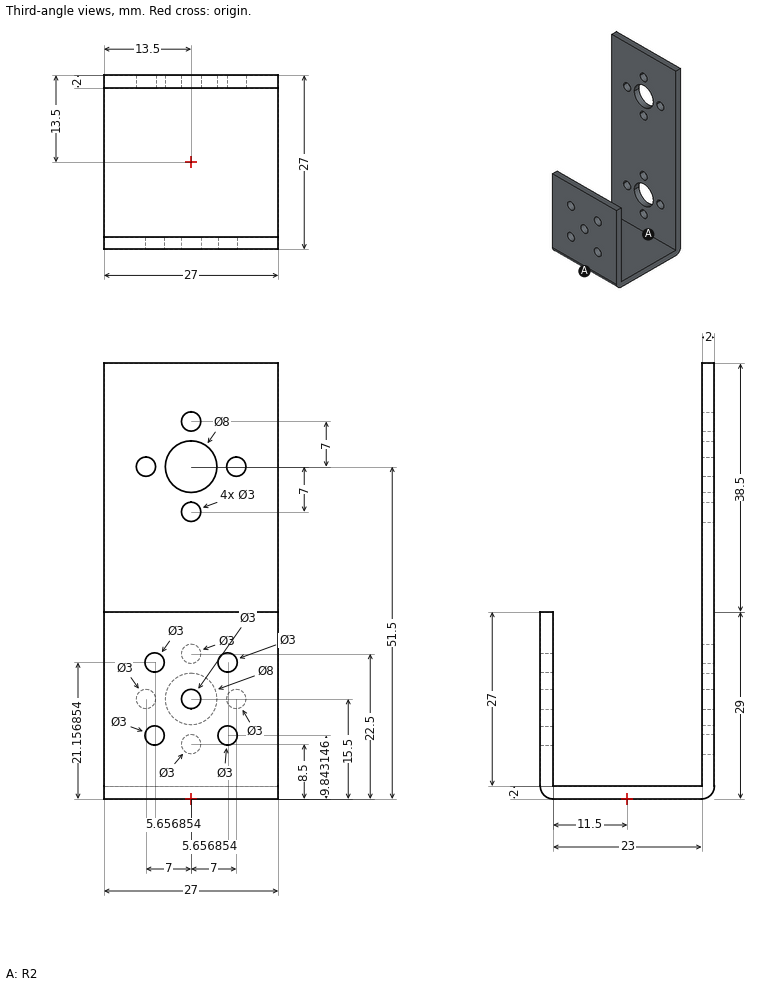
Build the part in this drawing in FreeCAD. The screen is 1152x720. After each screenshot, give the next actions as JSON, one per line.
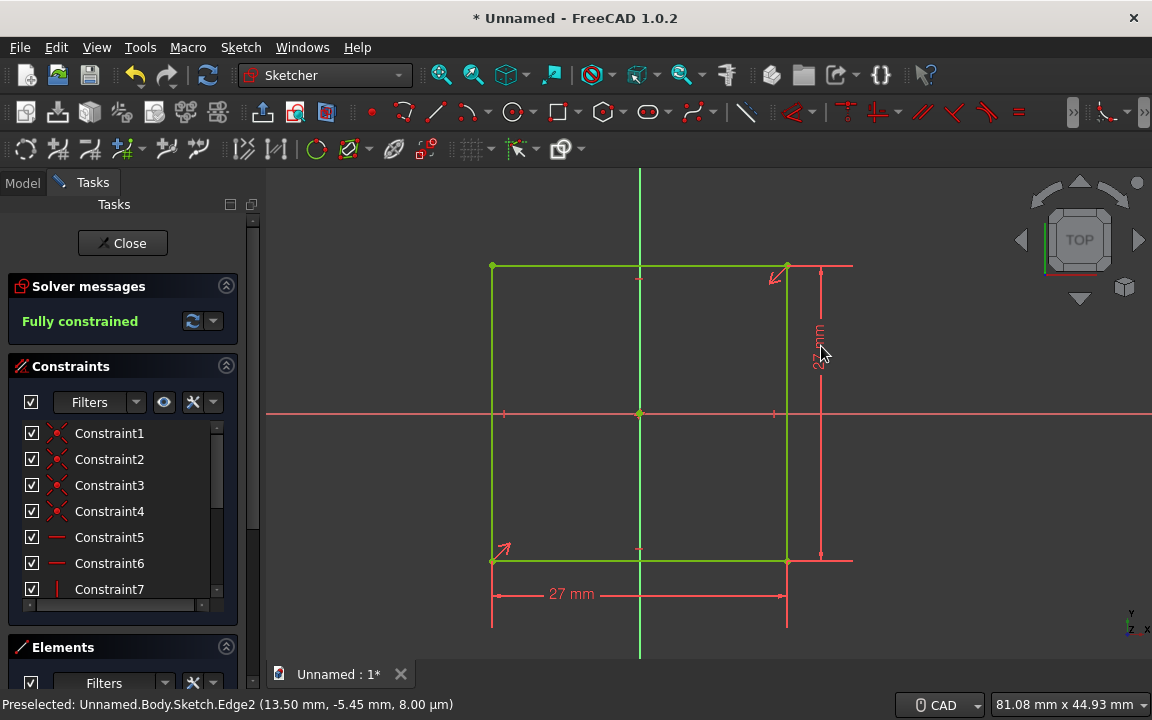
{"action": "left_click", "coordinate": [123, 243]}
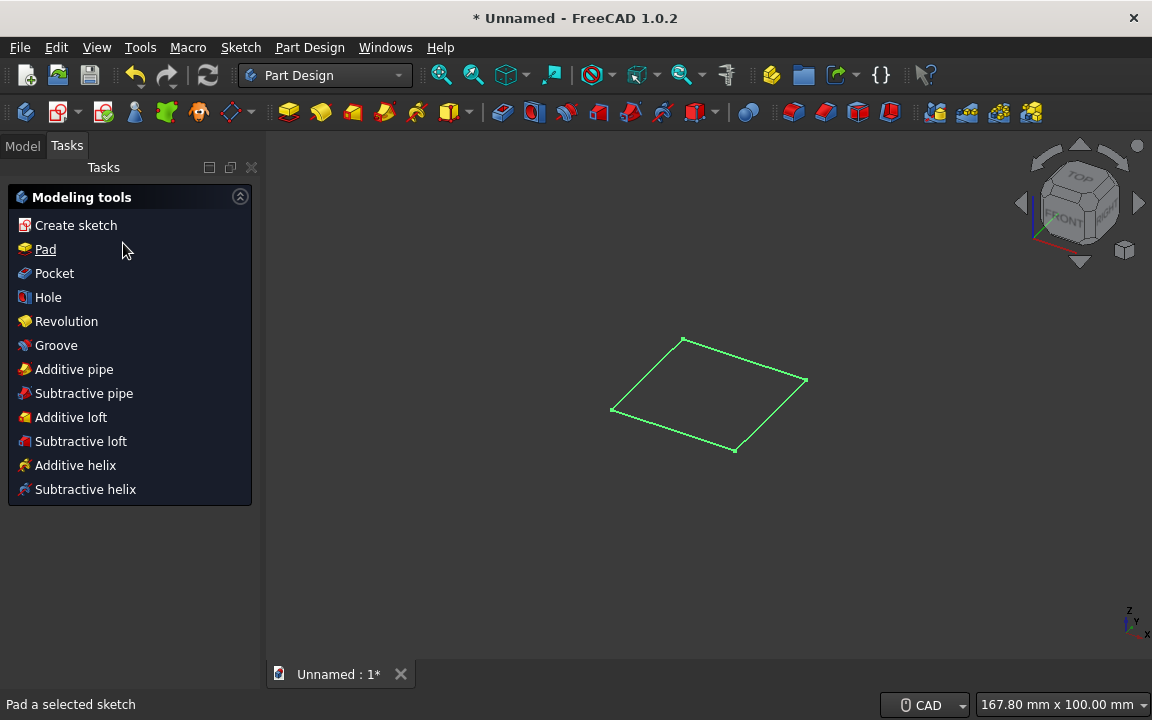
{"action": "left_click", "coordinate": [290, 112]}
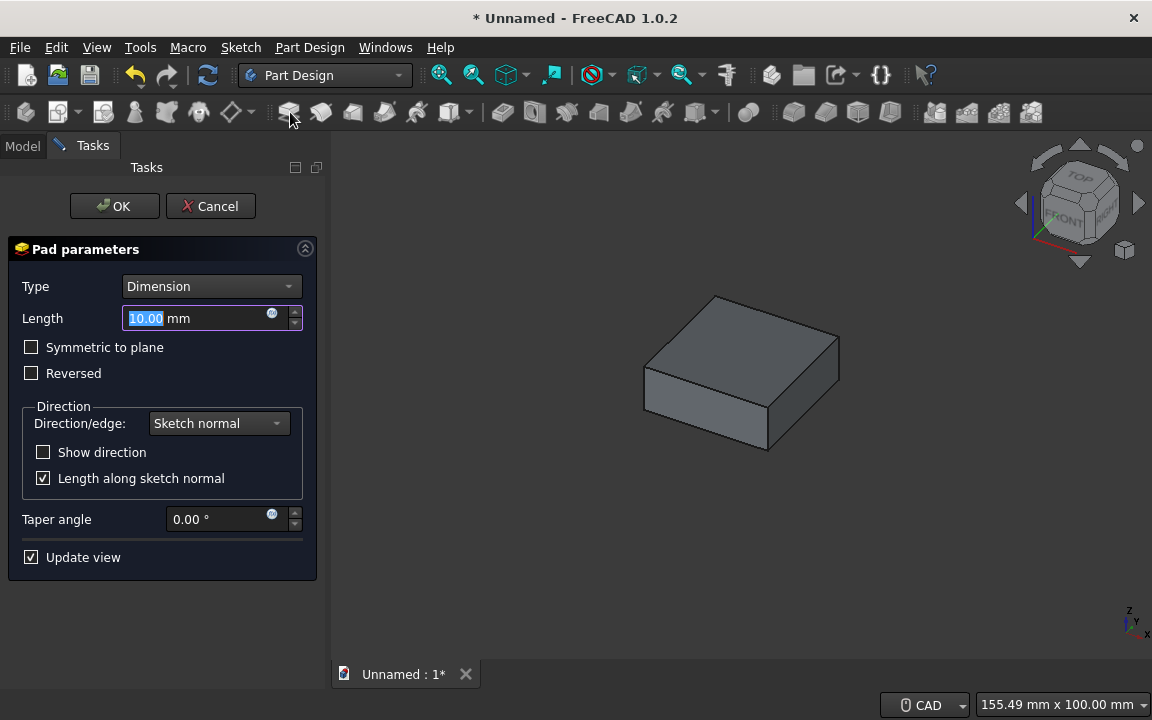
{"action": "type", "text": "29"}
{"action": "key", "text": "Tab"}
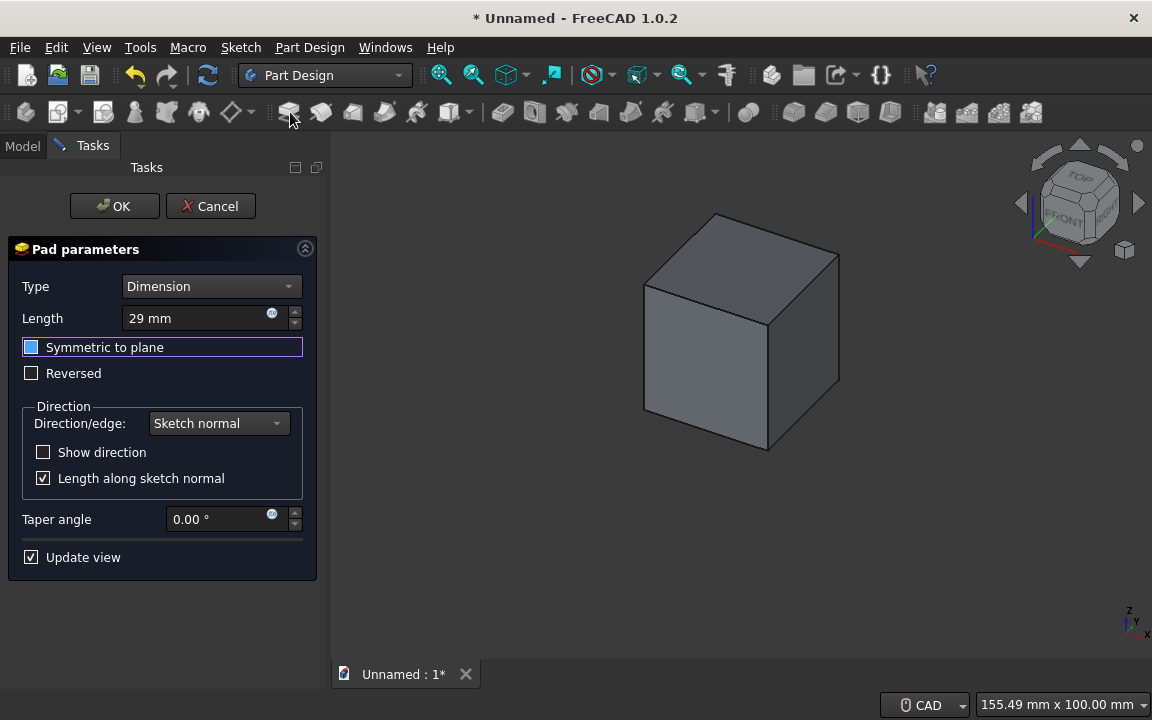
{"action": "left_click", "coordinate": [115, 206]}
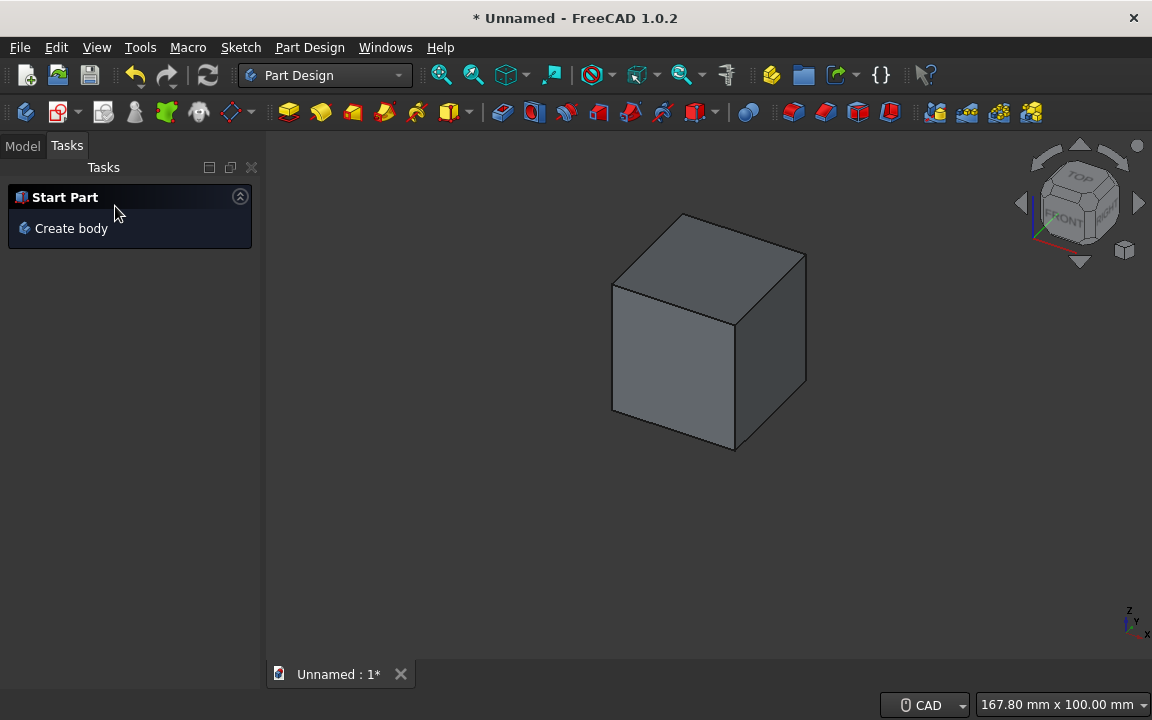
{"action": "left_click", "coordinate": [442, 76]}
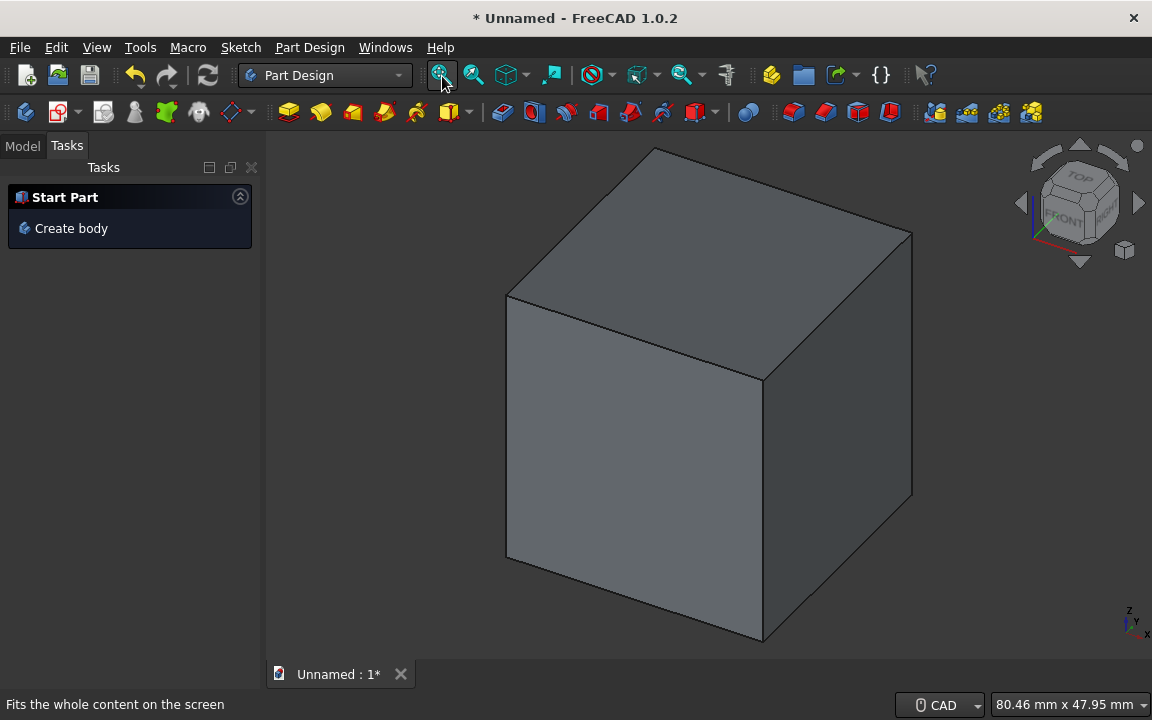
{"action": "left_click", "coordinate": [838, 437]}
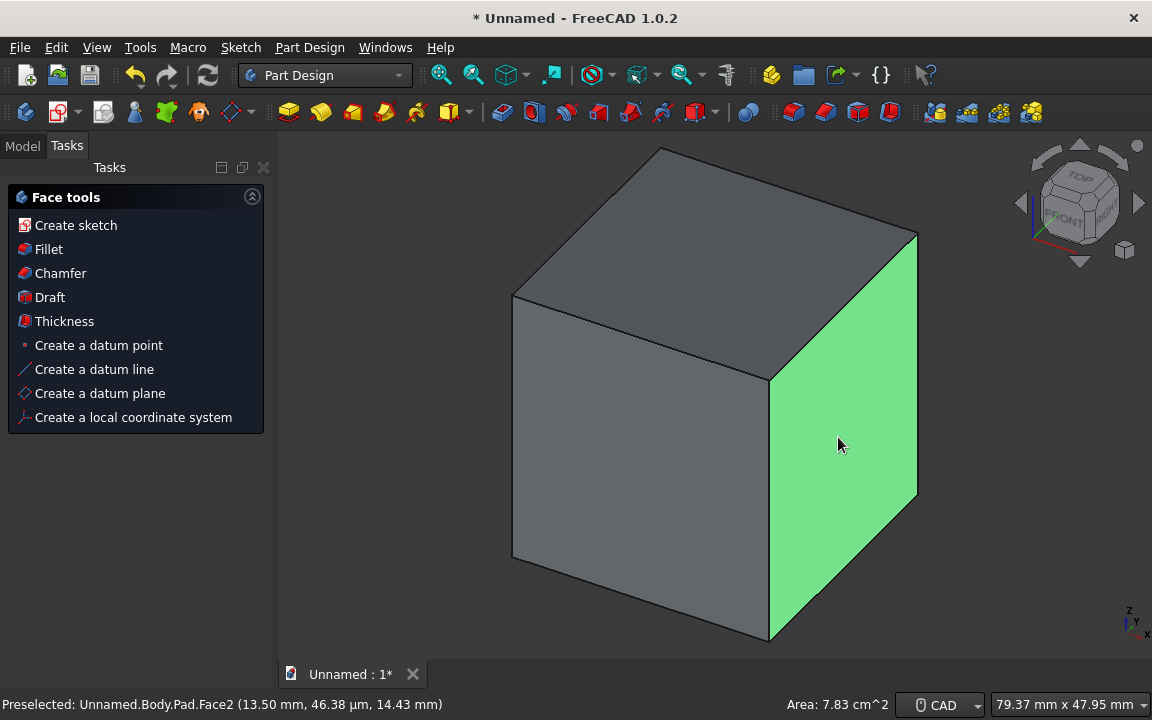
{"action": "left_click", "coordinate": [58, 112]}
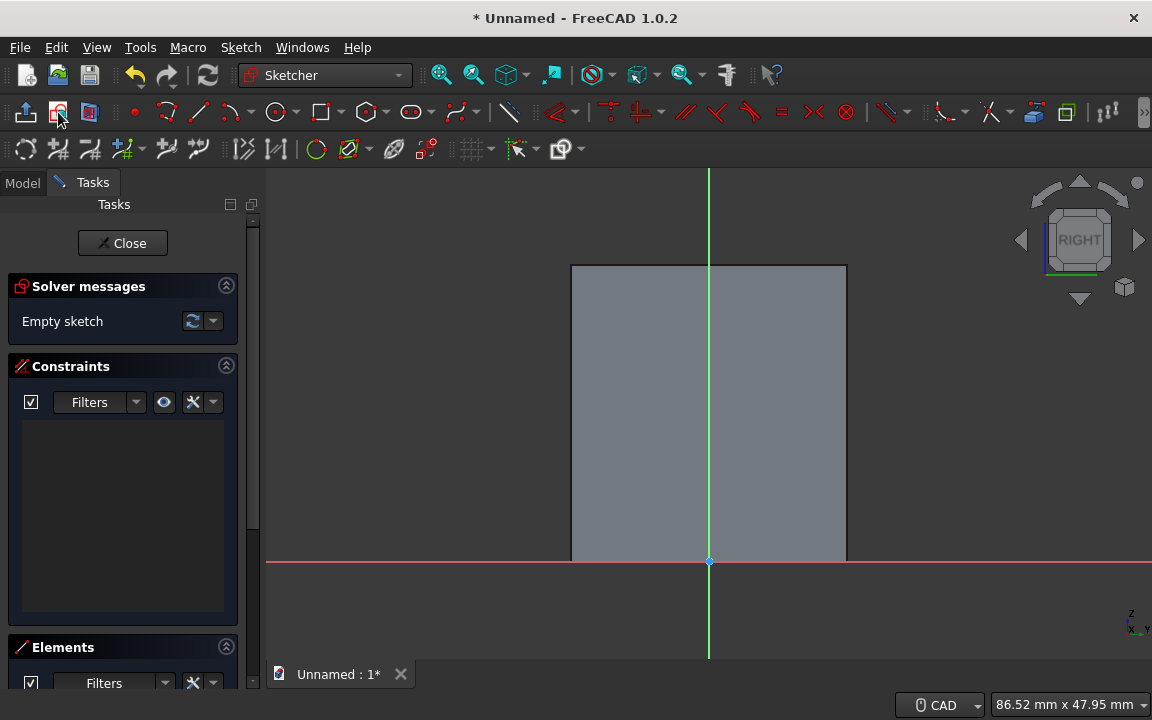
{"action": "key", "text": "g r"}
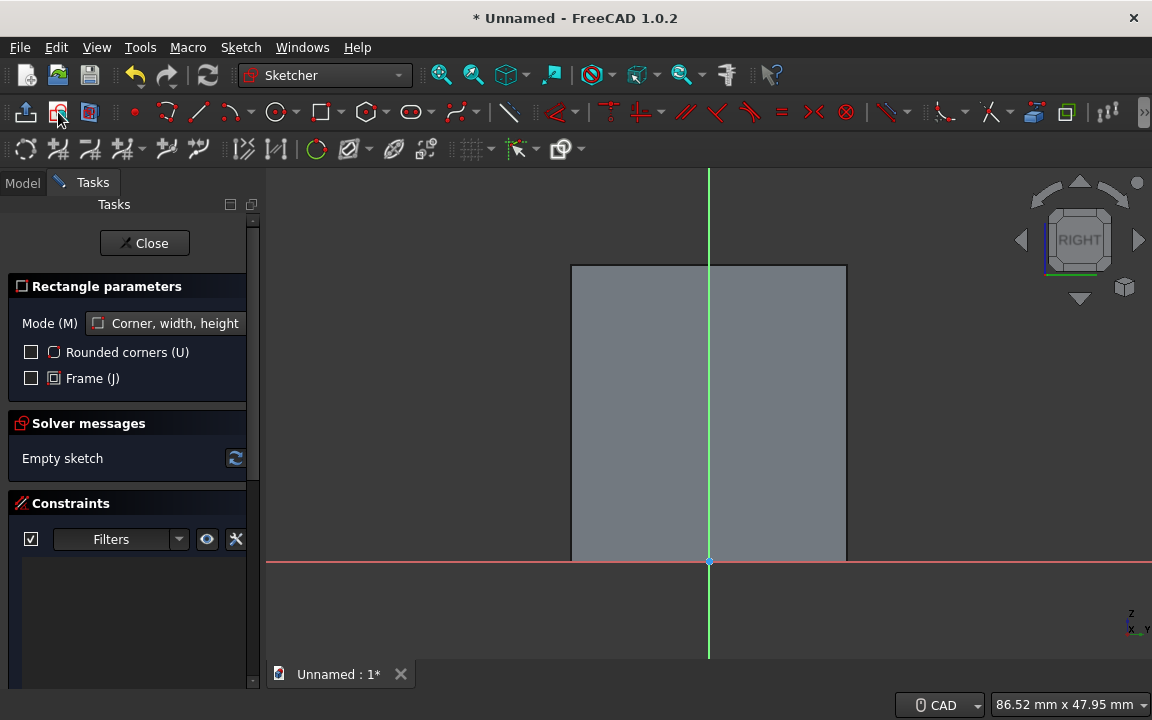
{"action": "left_click", "coordinate": [591, 265]}
{"action": "left_click", "coordinate": [827, 542]}
{"action": "key", "text": "Escape"}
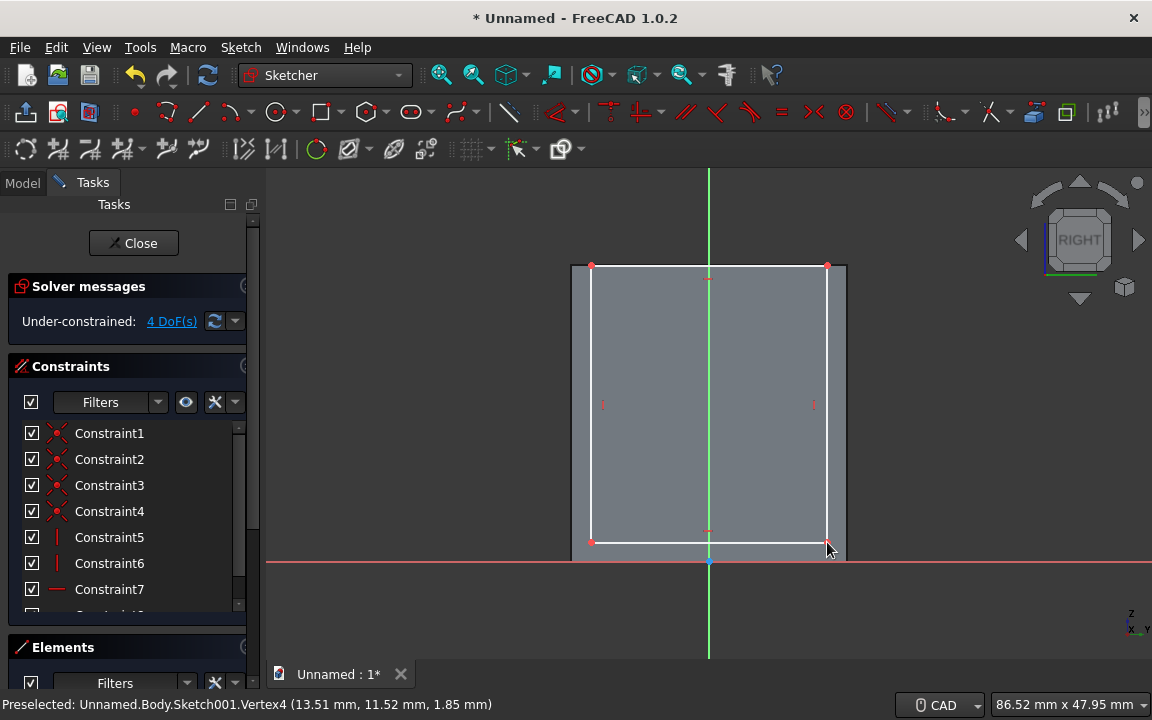
{"action": "left_click", "coordinate": [556, 112]}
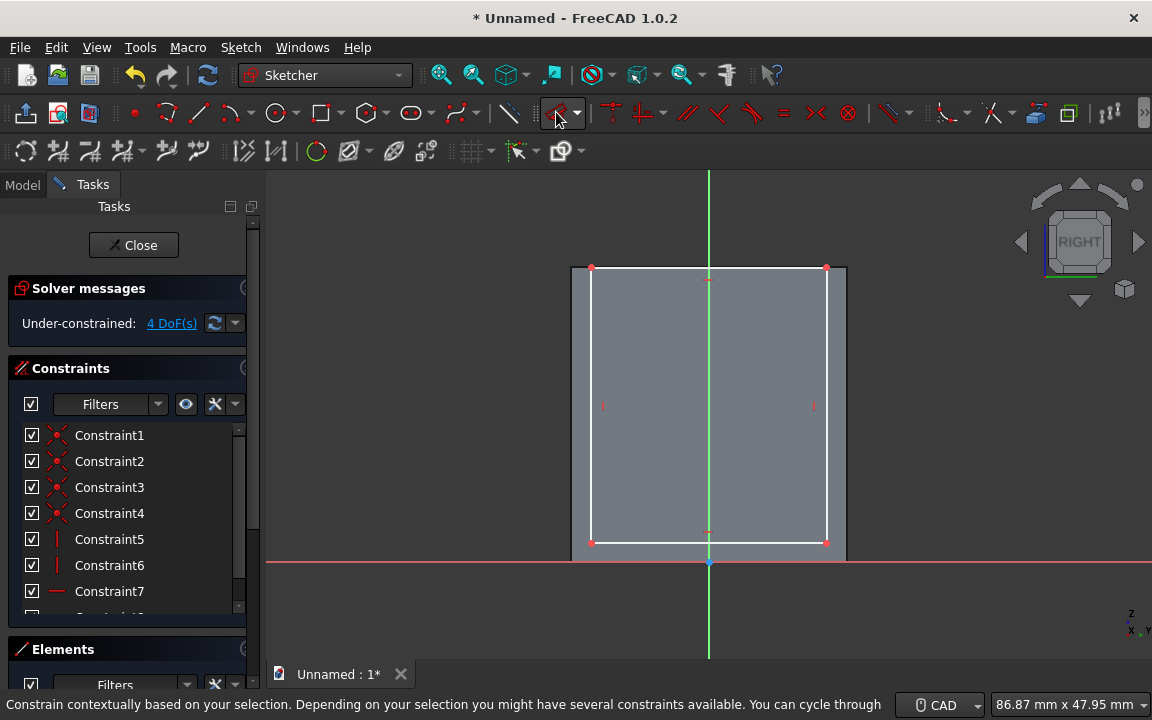
{"action": "left_click", "coordinate": [591, 350]}
{"action": "left_click", "coordinate": [557, 406]}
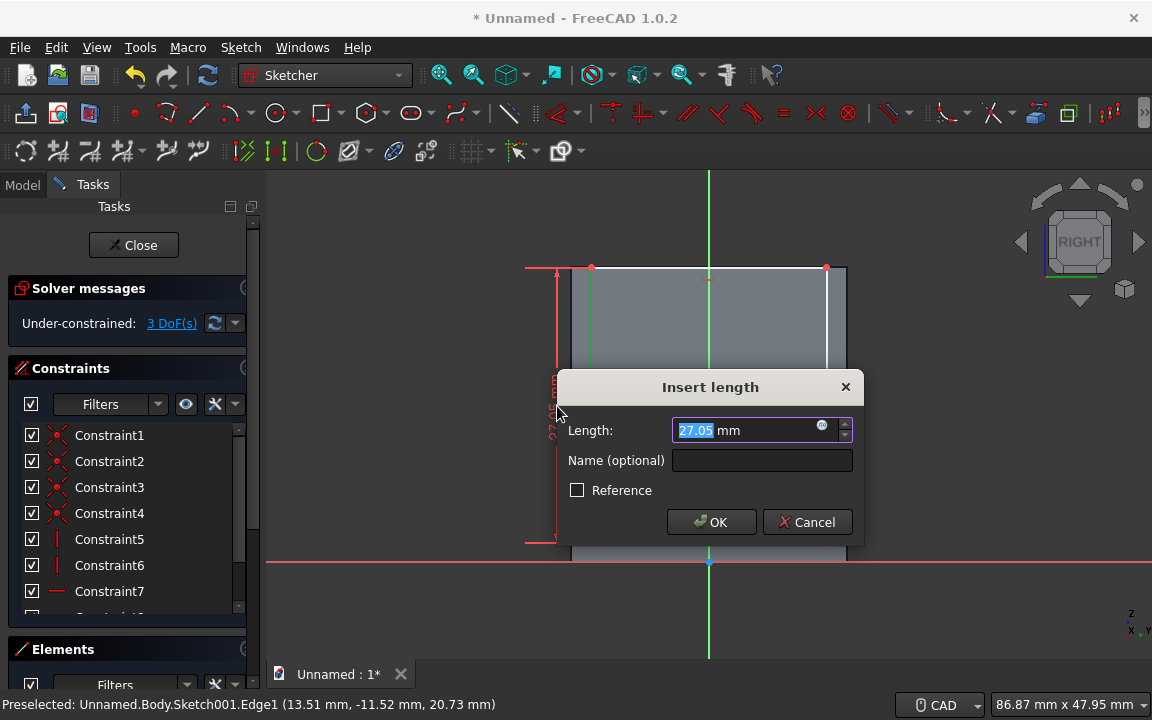
{"action": "type", "text": "27"}
{"action": "key", "text": "Return"}